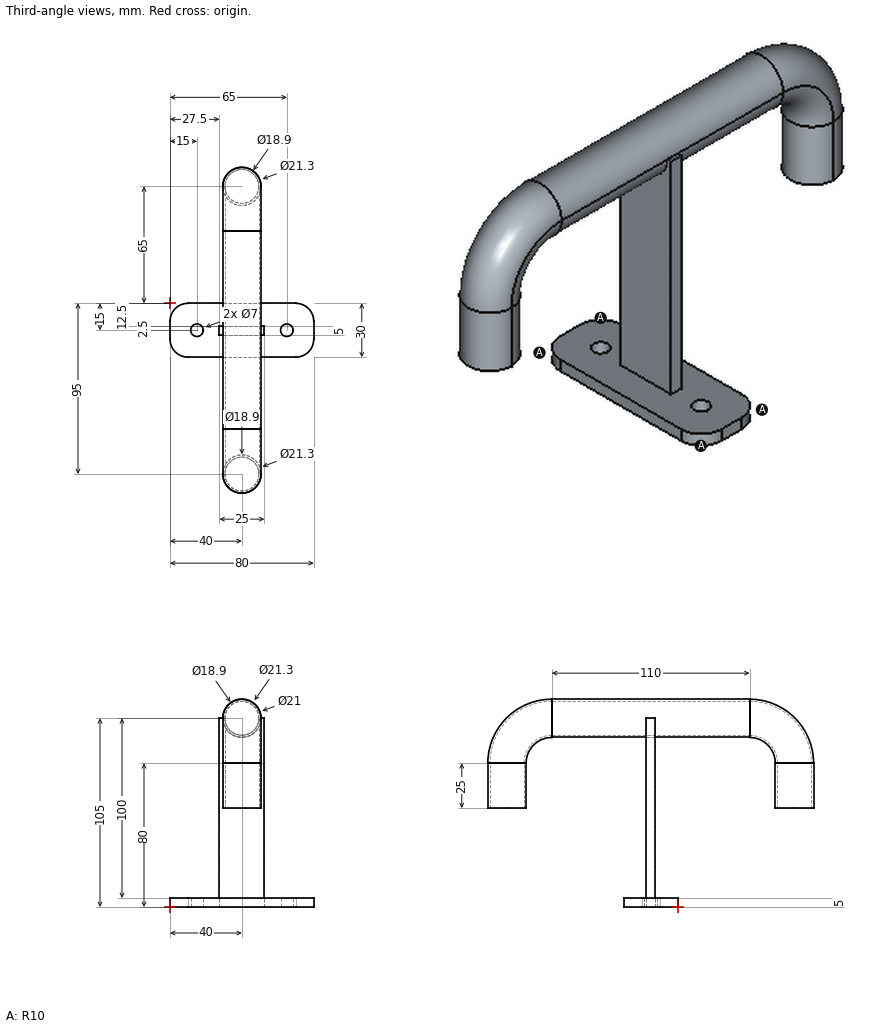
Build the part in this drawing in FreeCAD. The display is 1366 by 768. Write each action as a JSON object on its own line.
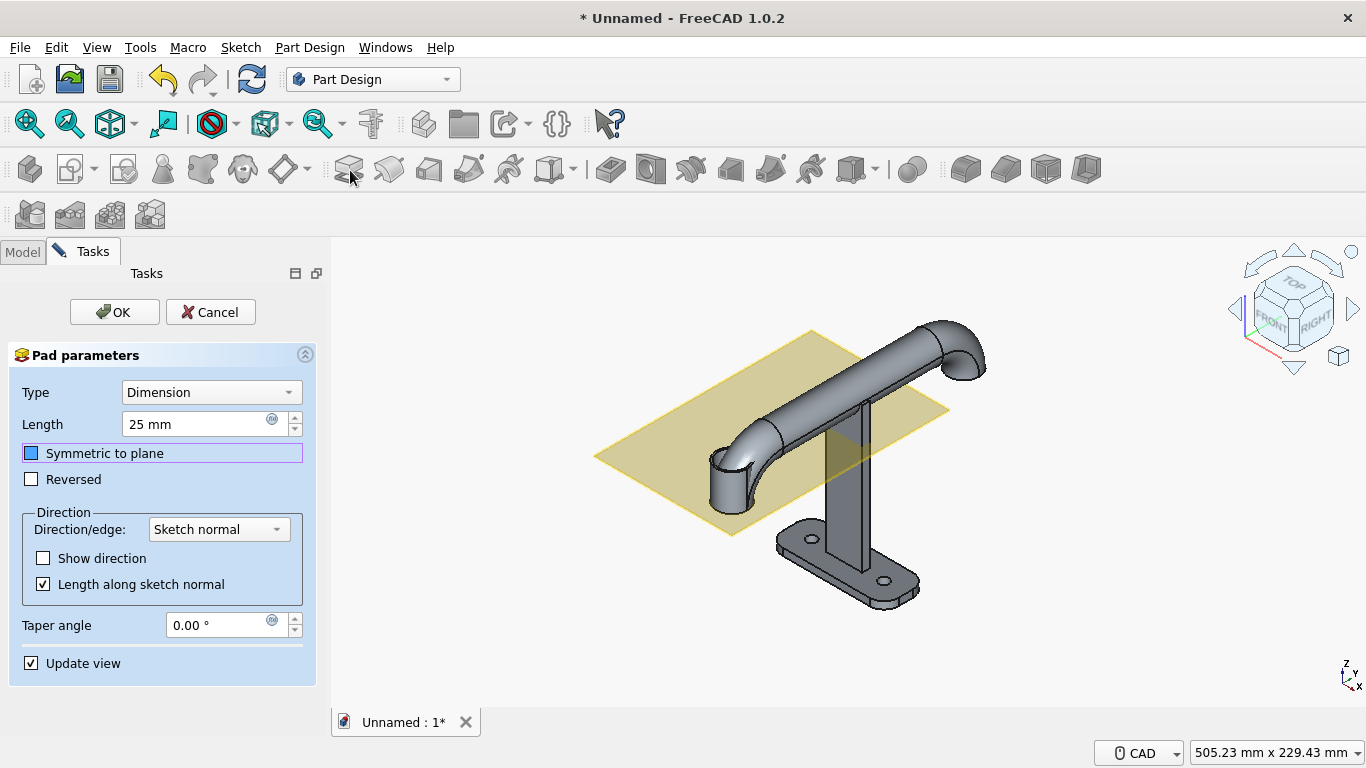
{"action": "left_click", "coordinate": [30, 479]}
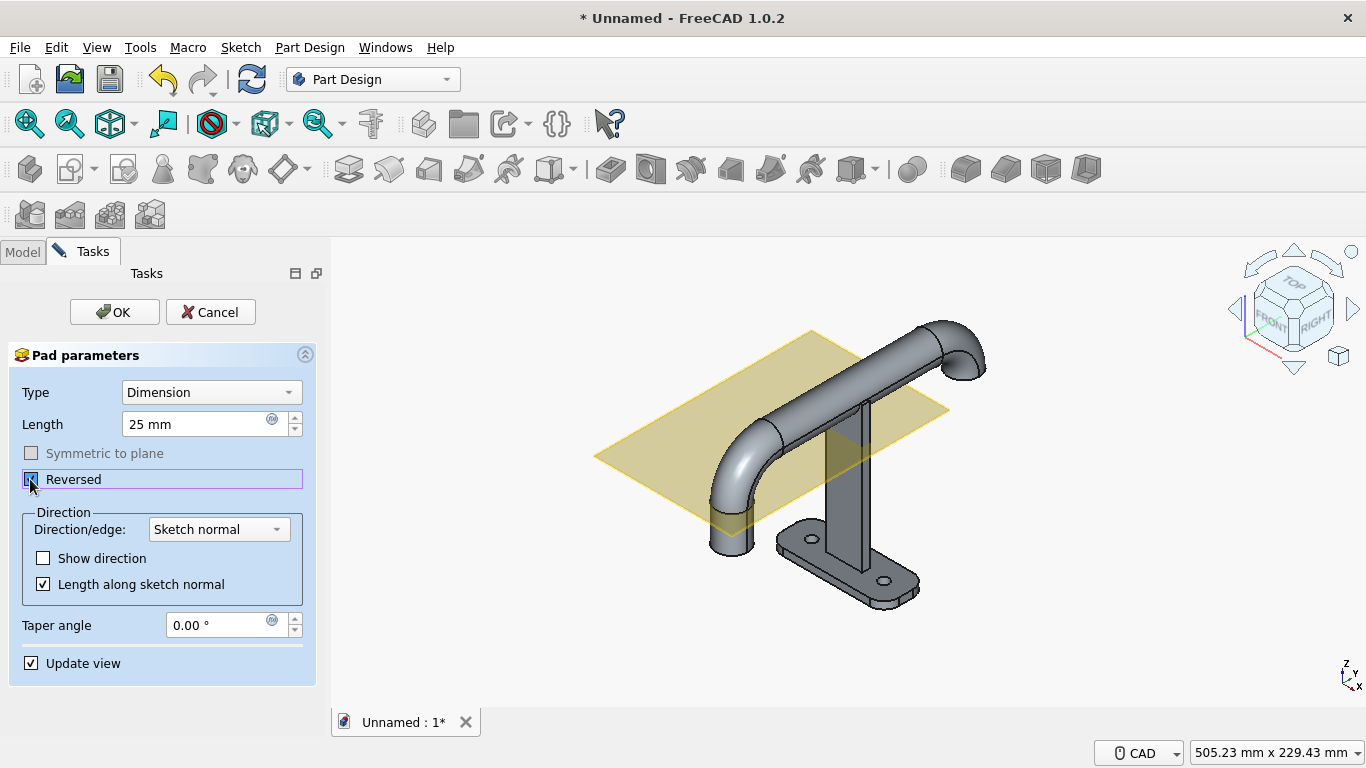
{"action": "left_click", "coordinate": [115, 312]}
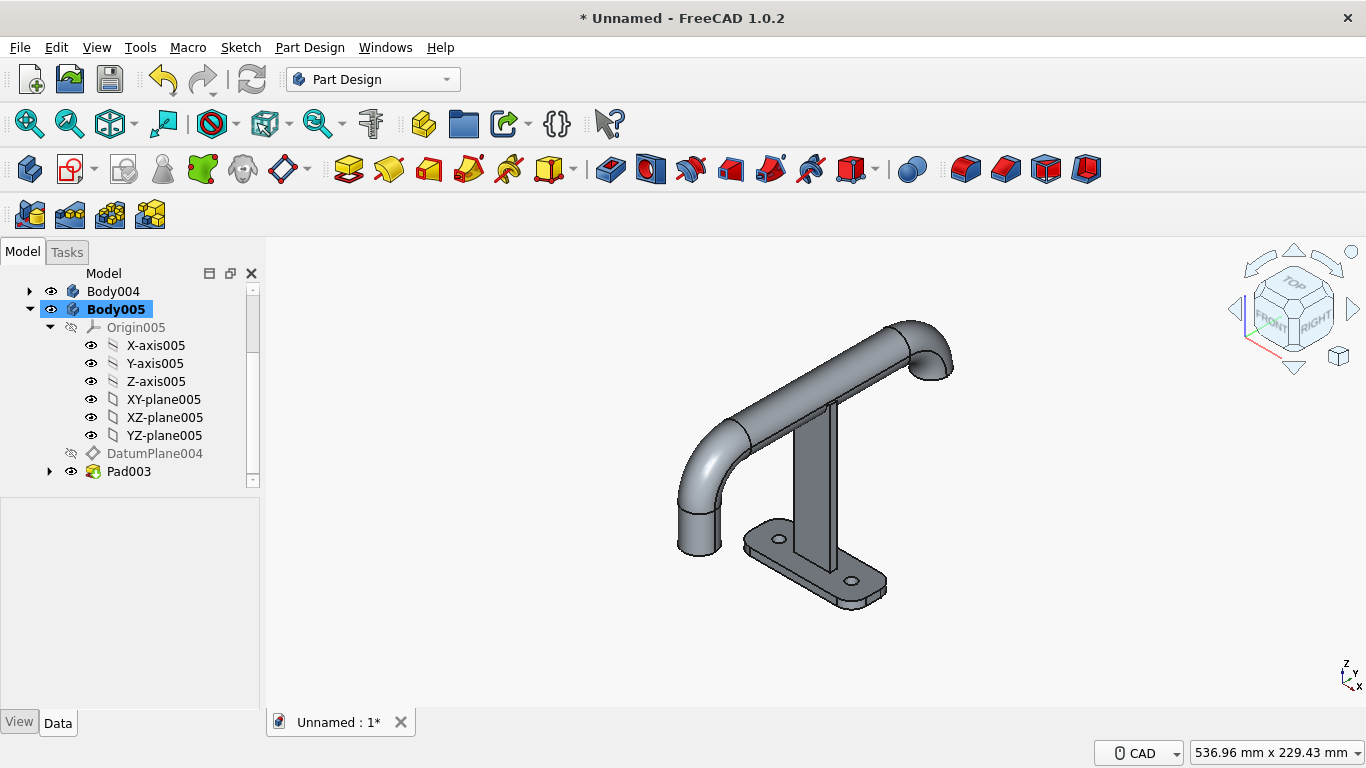
{"action": "left_click", "coordinate": [30, 124]}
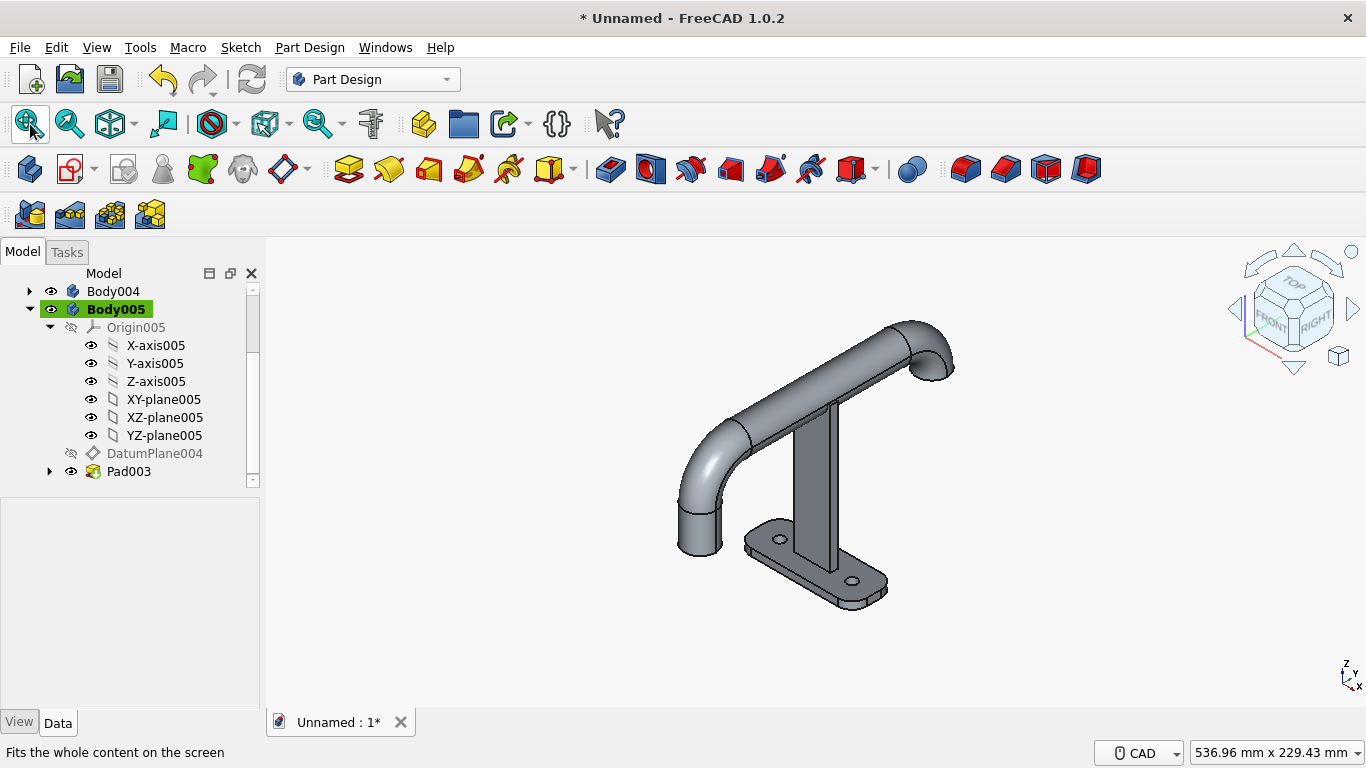
{"action": "left_click", "coordinate": [30, 170]}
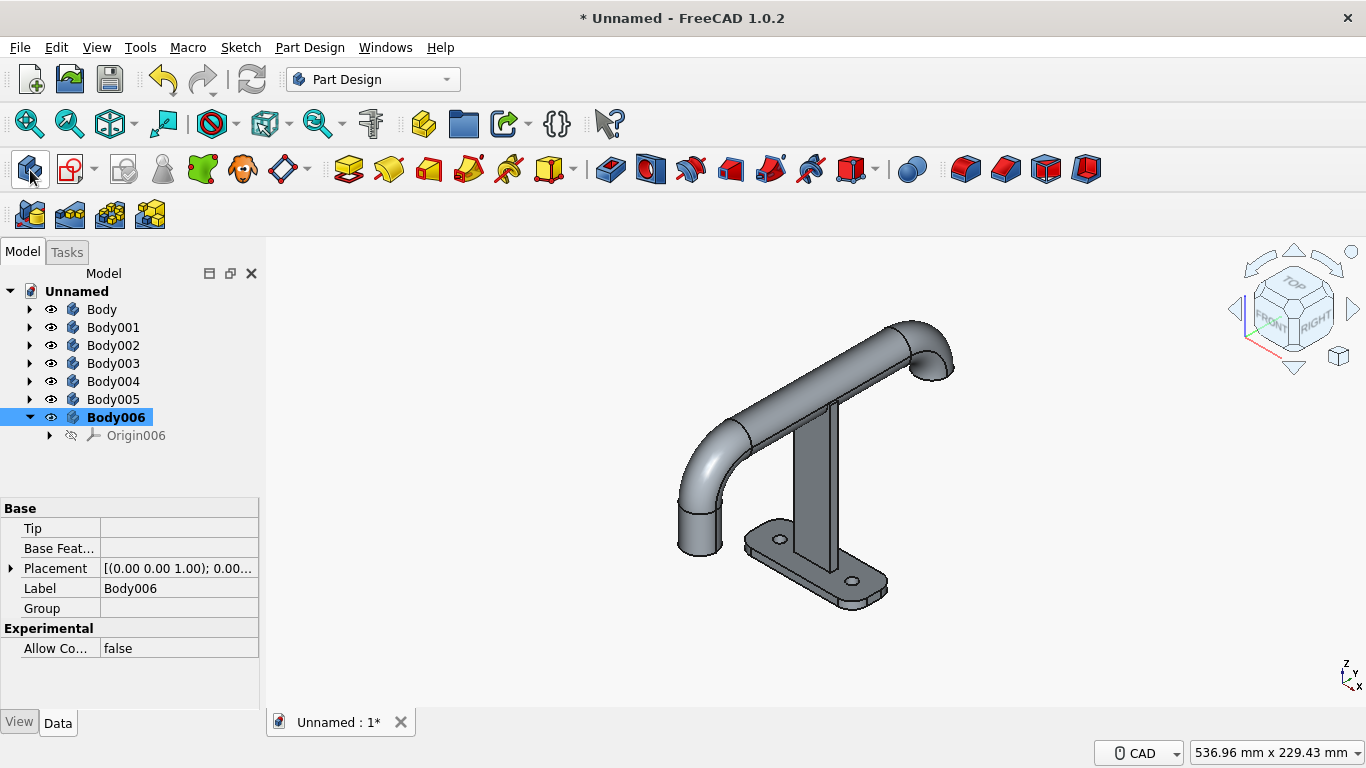
{"action": "left_click", "coordinate": [50, 435]}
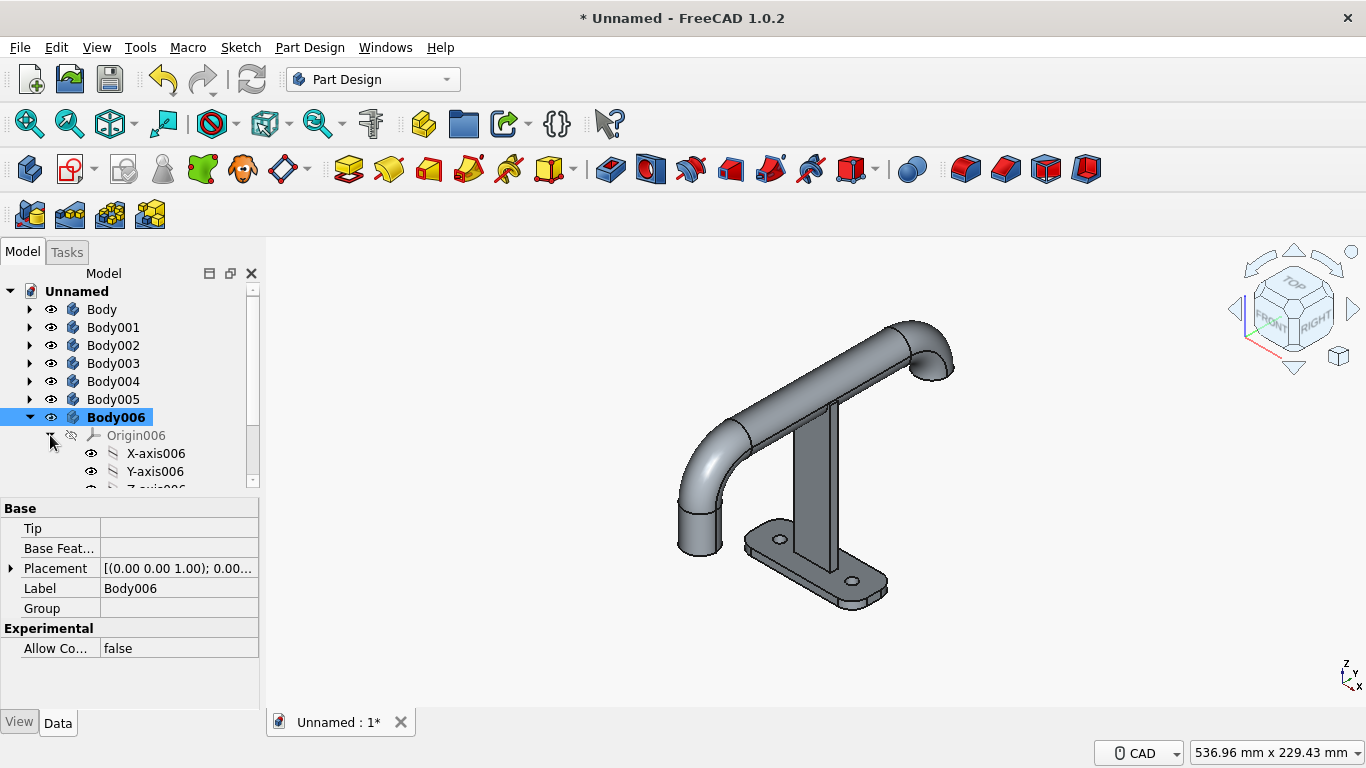
{"action": "scroll", "coordinate": [100, 377], "scroll_direction": "down", "scroll_amount": 3}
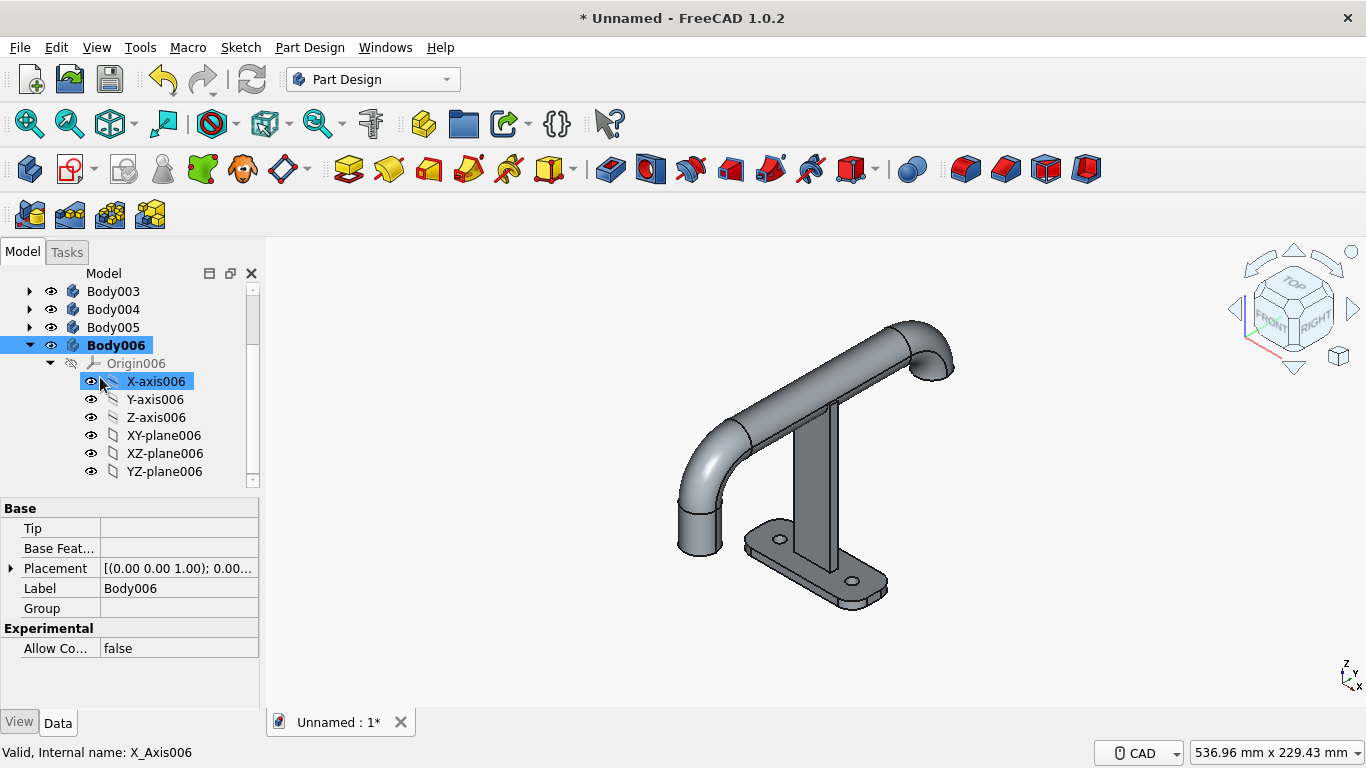
{"action": "left_click", "coordinate": [136, 435]}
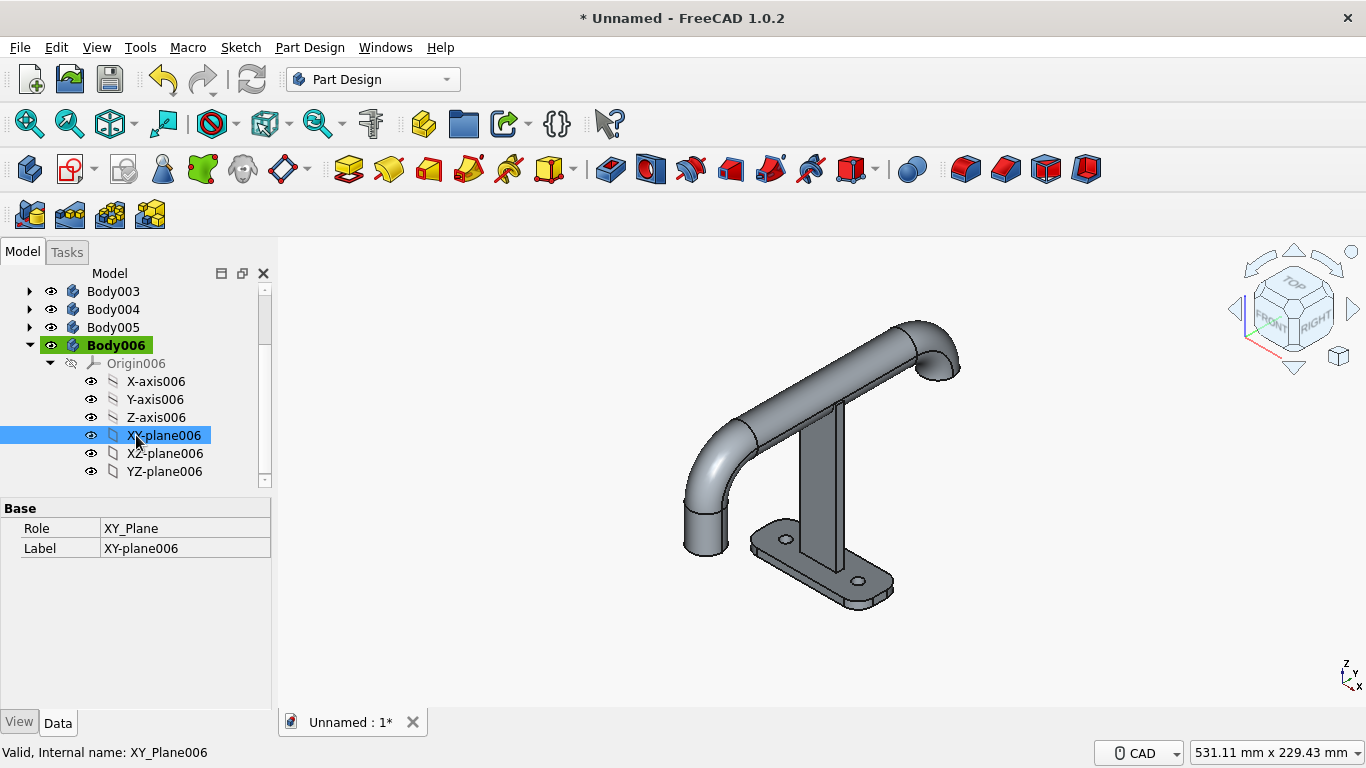
{"action": "left_click", "coordinate": [284, 170]}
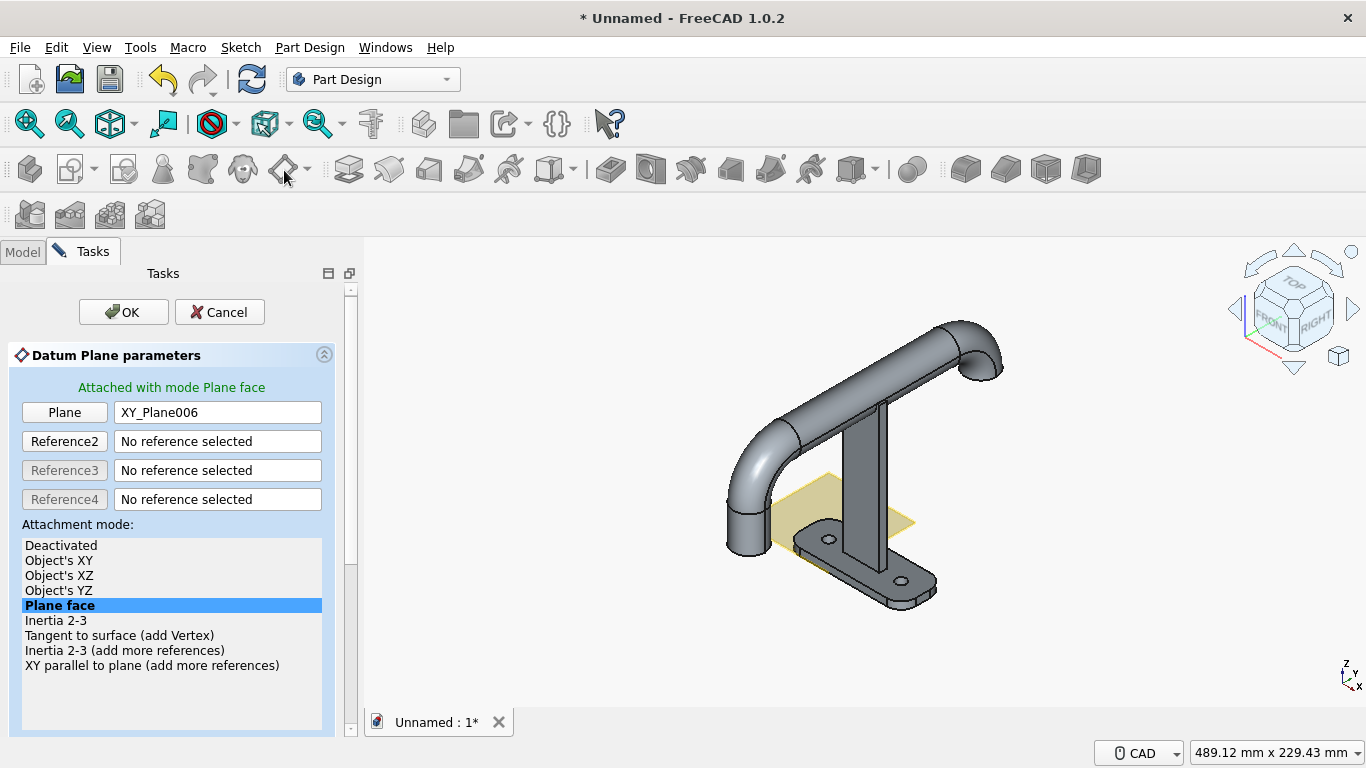
{"action": "scroll", "coordinate": [351, 510], "scroll_direction": "down", "scroll_amount": 3}